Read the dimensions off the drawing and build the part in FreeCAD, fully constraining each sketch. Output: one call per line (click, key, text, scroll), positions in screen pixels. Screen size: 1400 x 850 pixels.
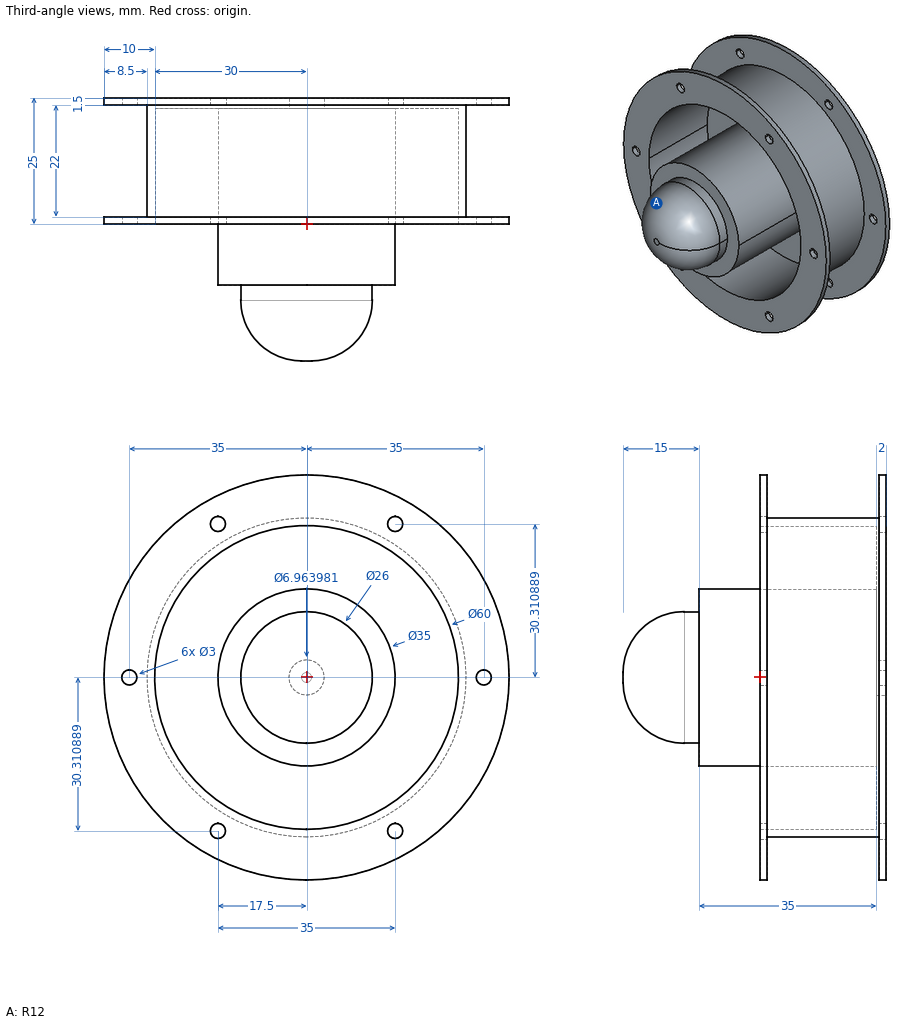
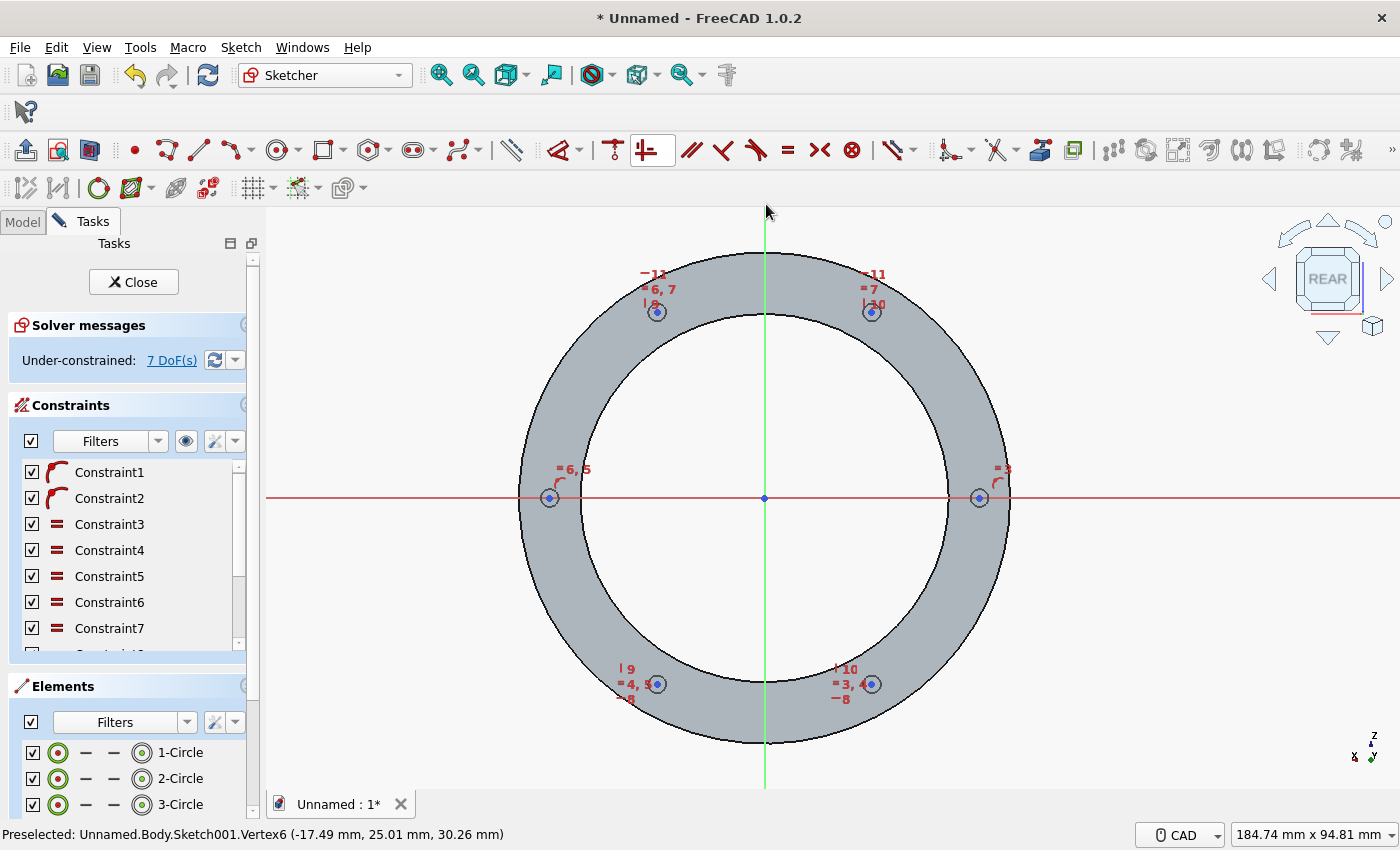
click(558, 150)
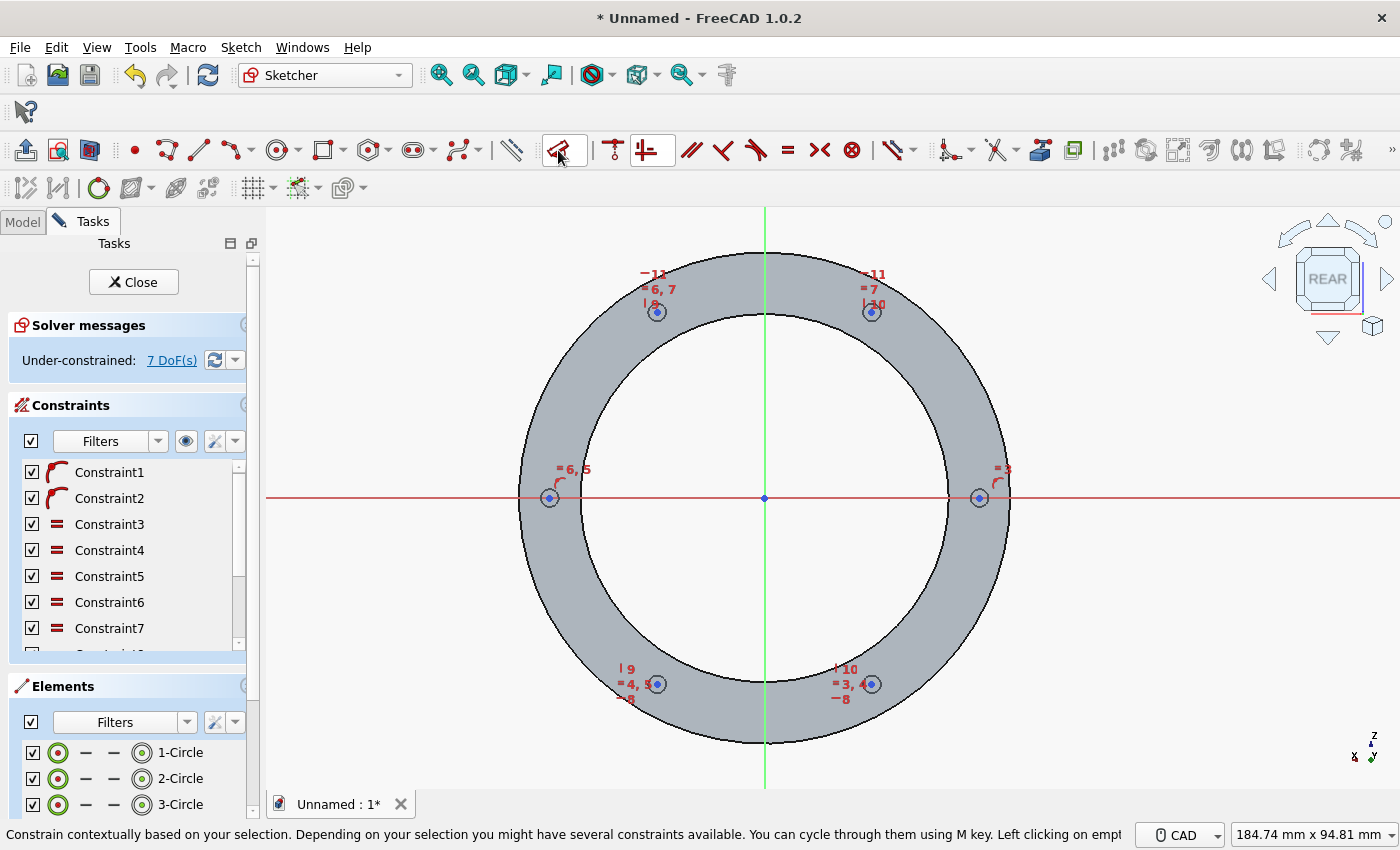
scroll(971, 498, up, 4)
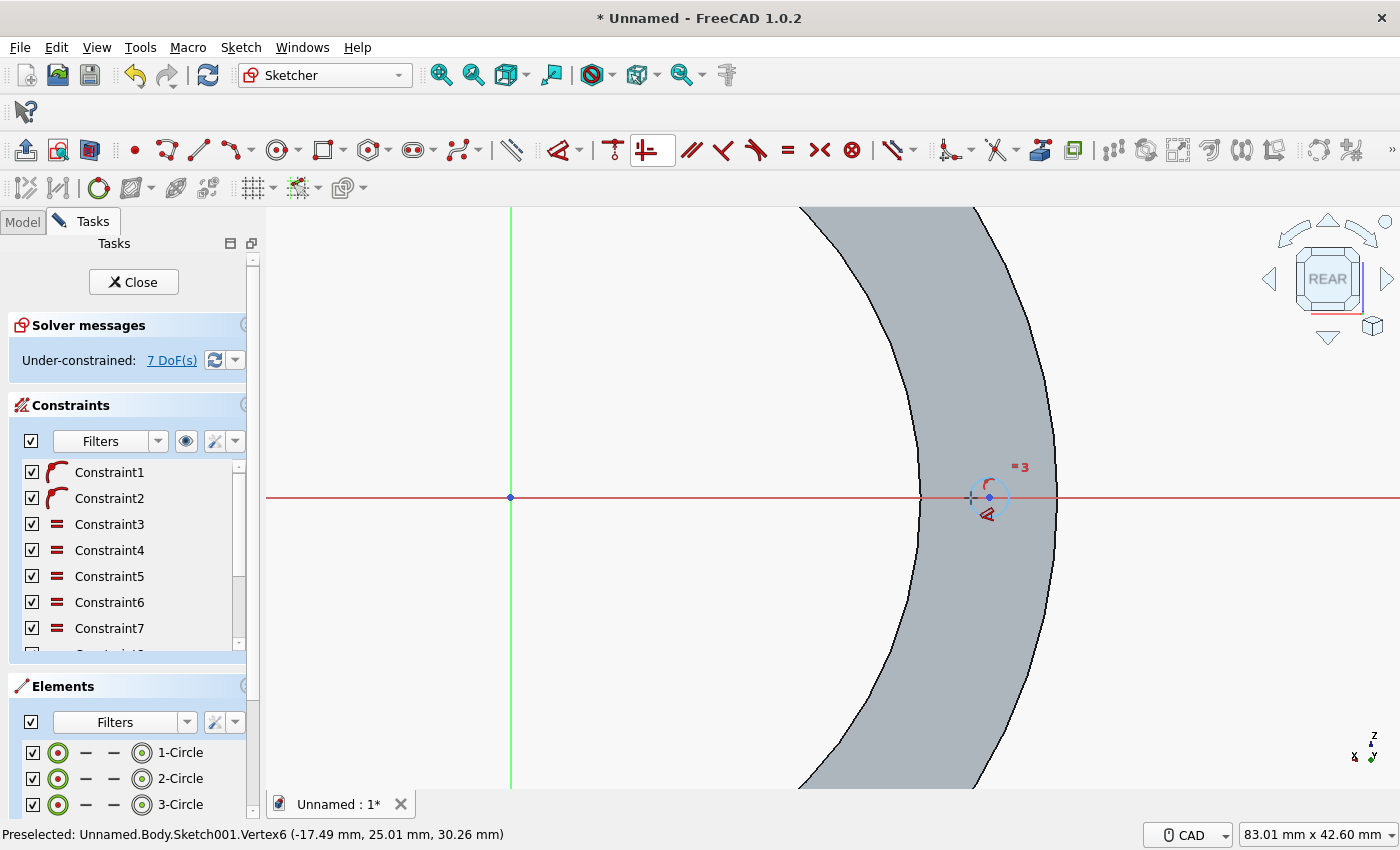
click(970, 497)
click(945, 472)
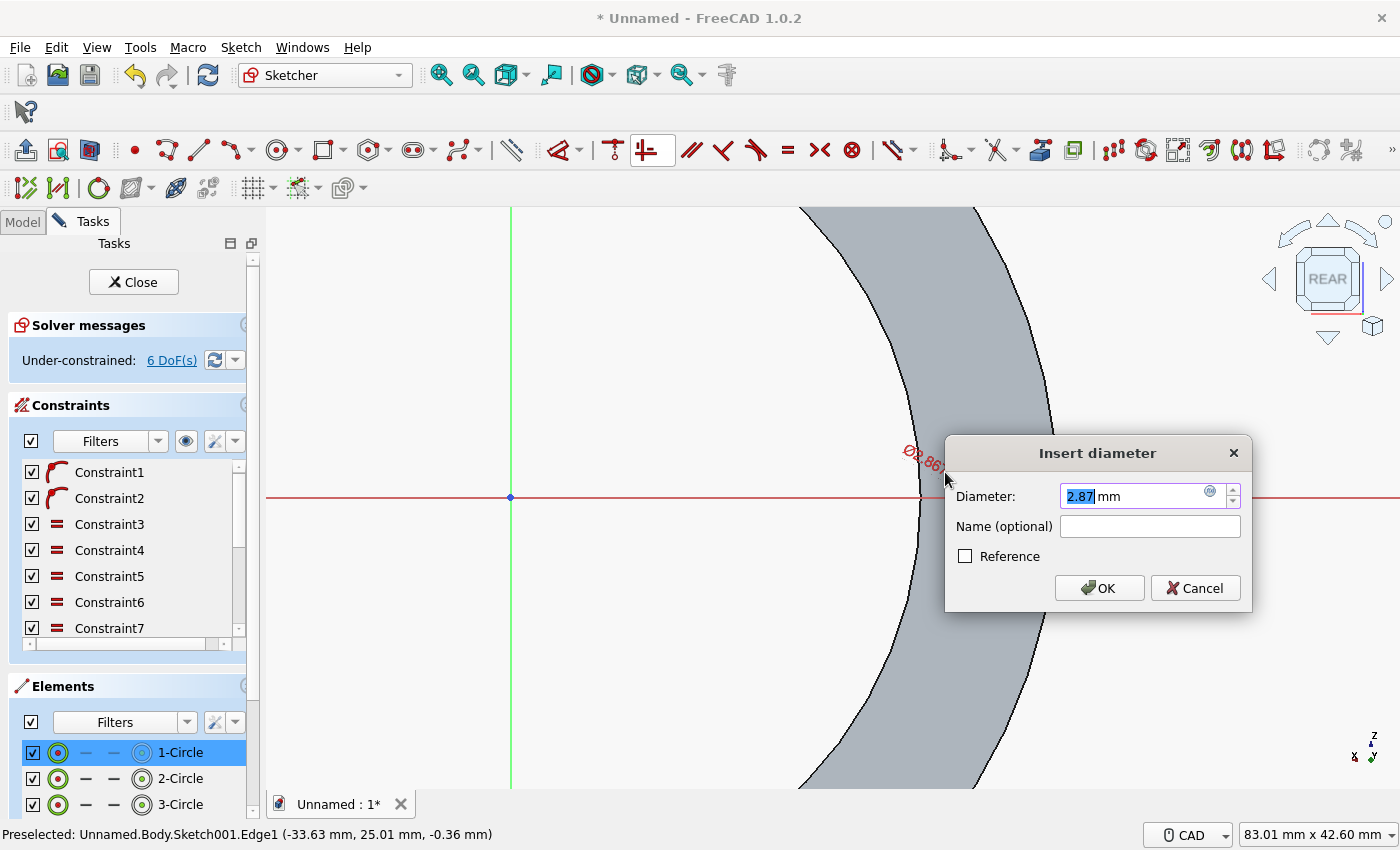
text(3)
key(Return)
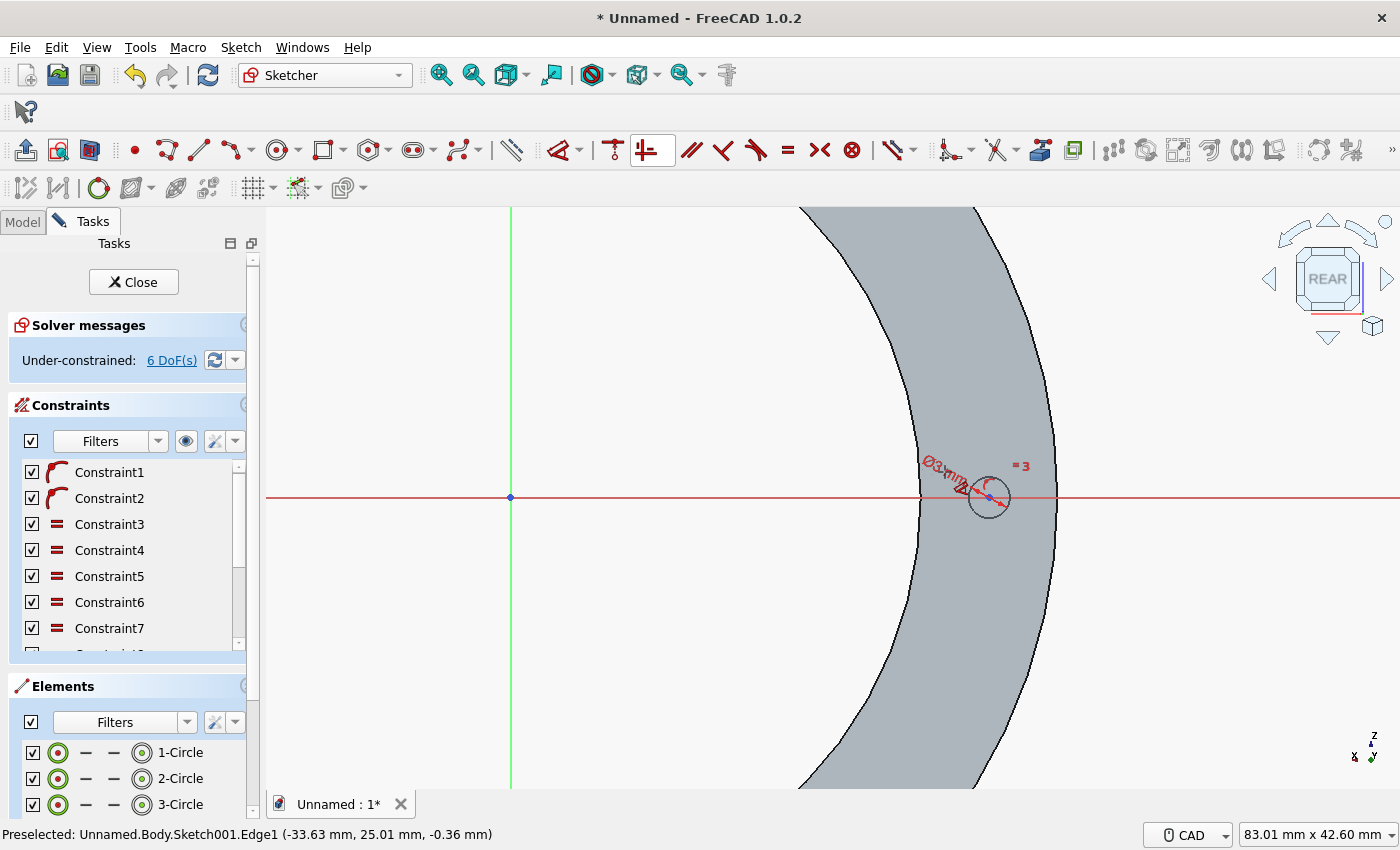
click(989, 498)
click(750, 532)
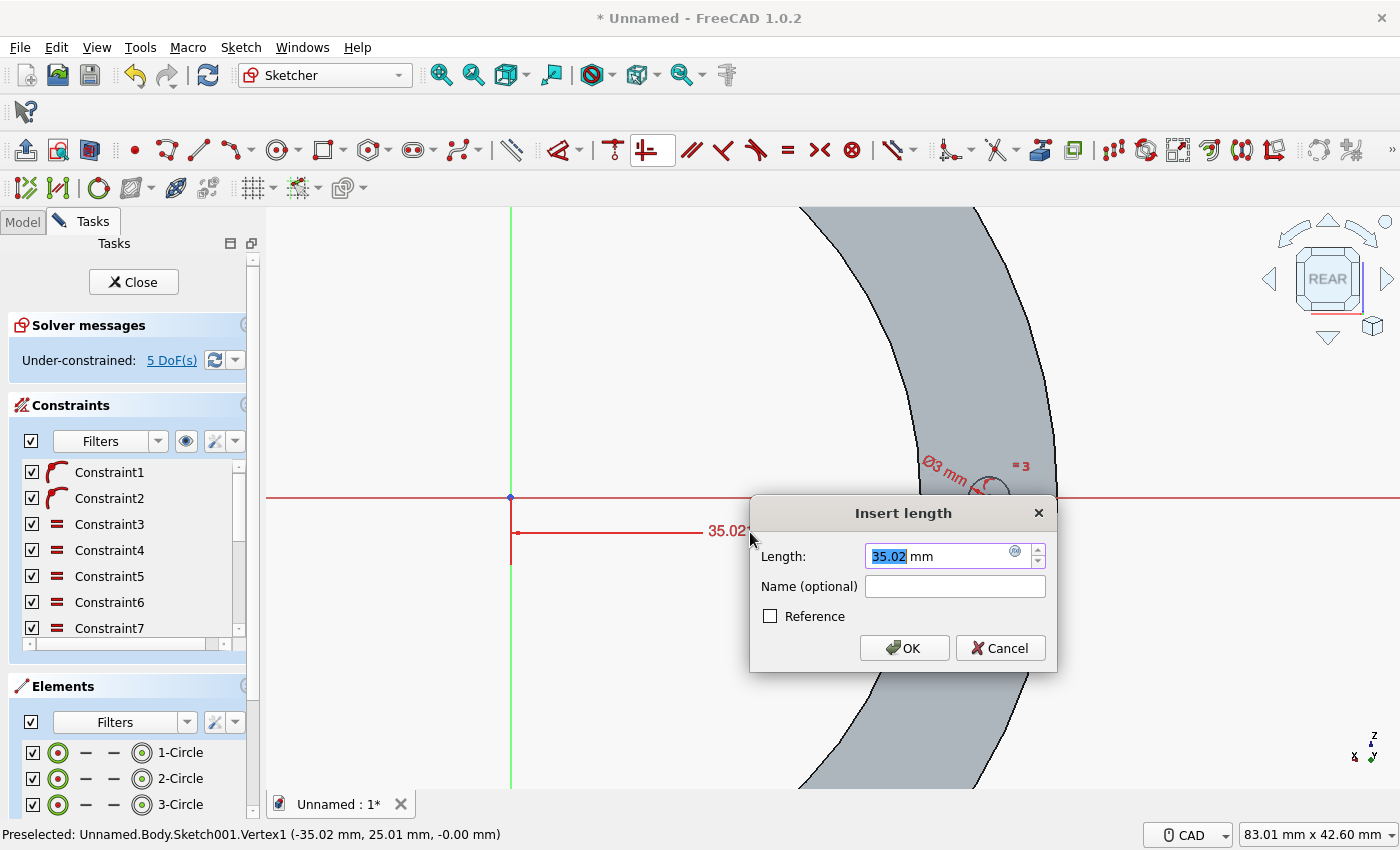
text(35)
key(Return)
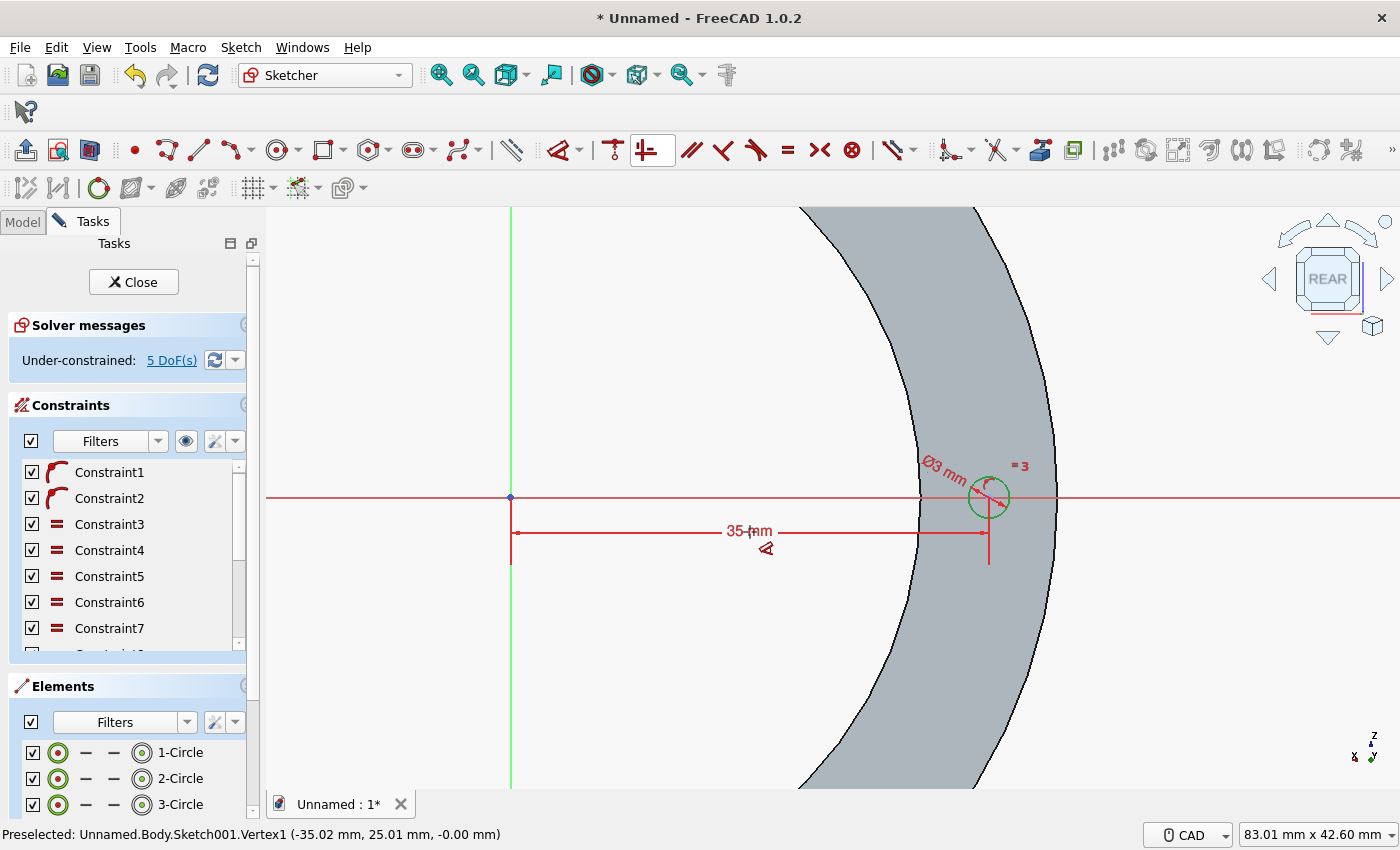
scroll(971, 498, down, 4)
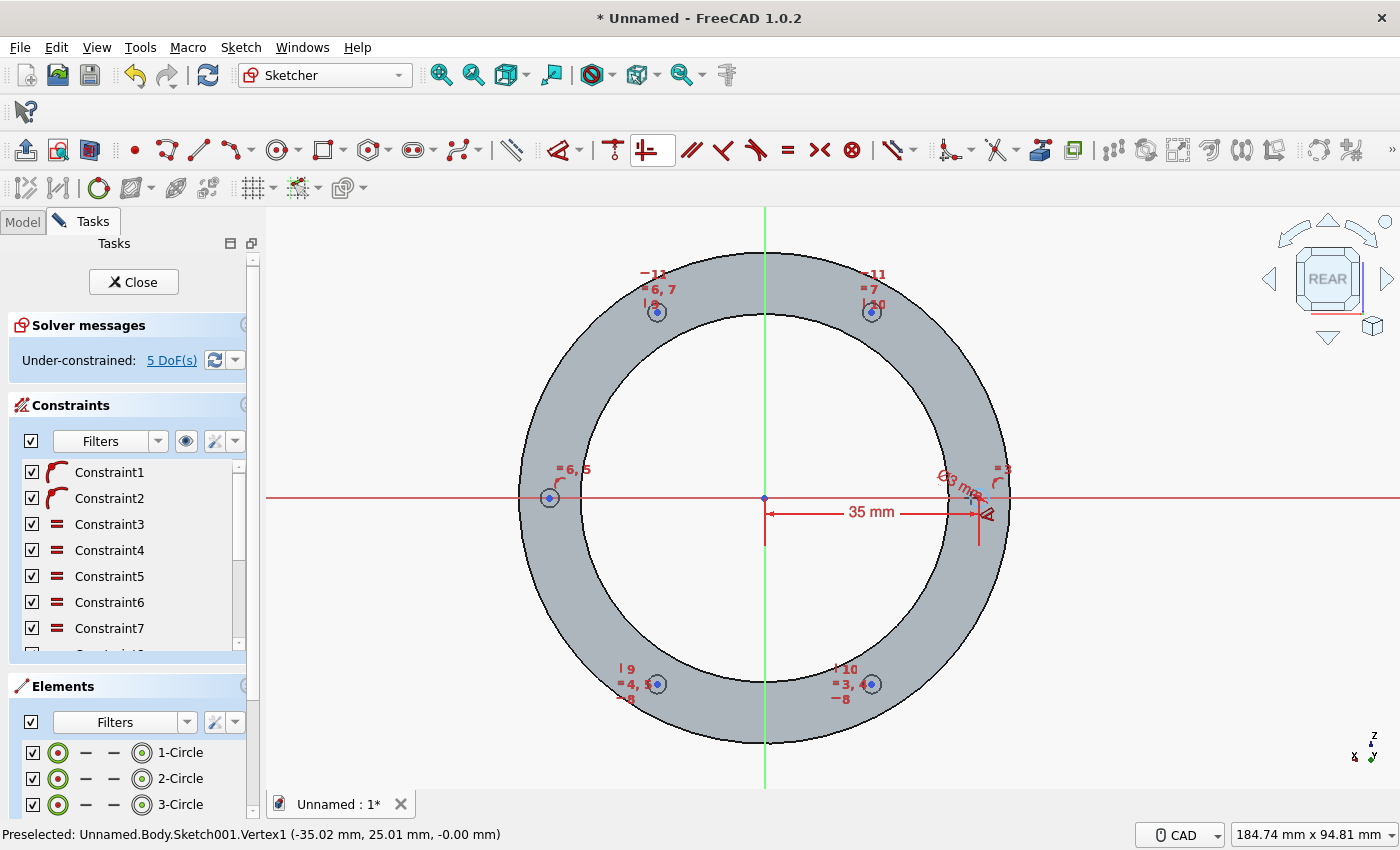
click(550, 498)
click(657, 532)